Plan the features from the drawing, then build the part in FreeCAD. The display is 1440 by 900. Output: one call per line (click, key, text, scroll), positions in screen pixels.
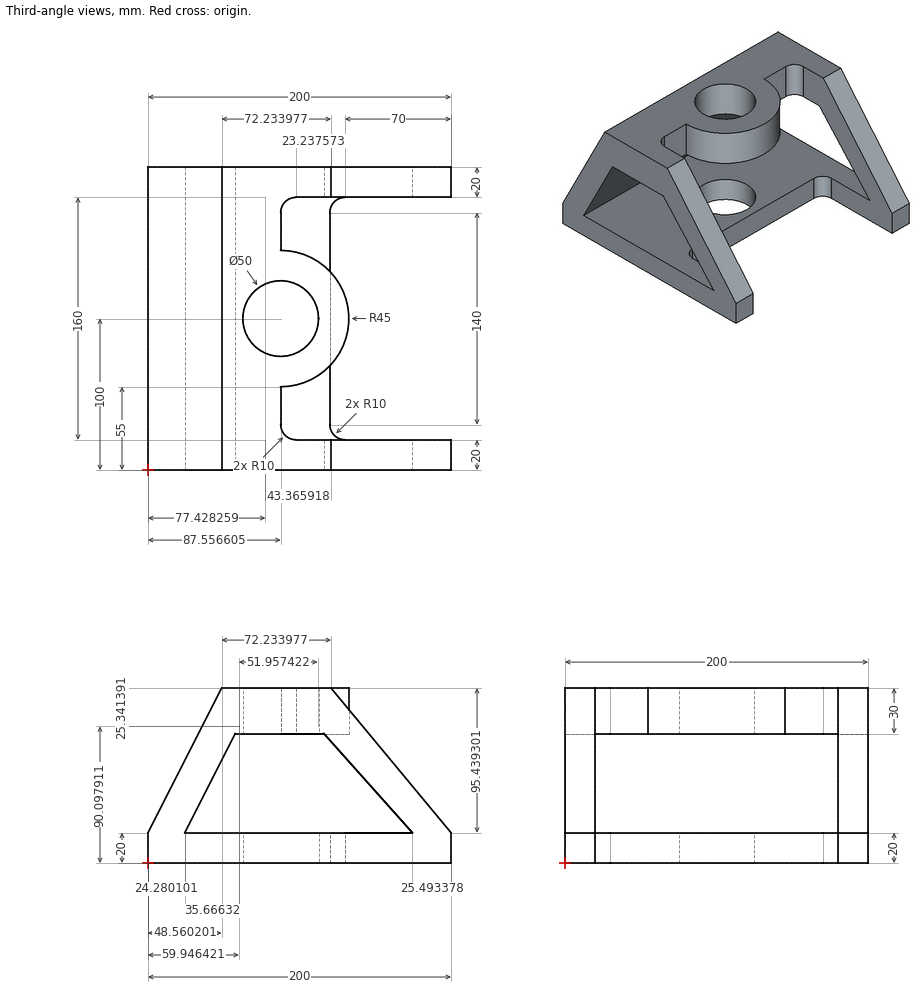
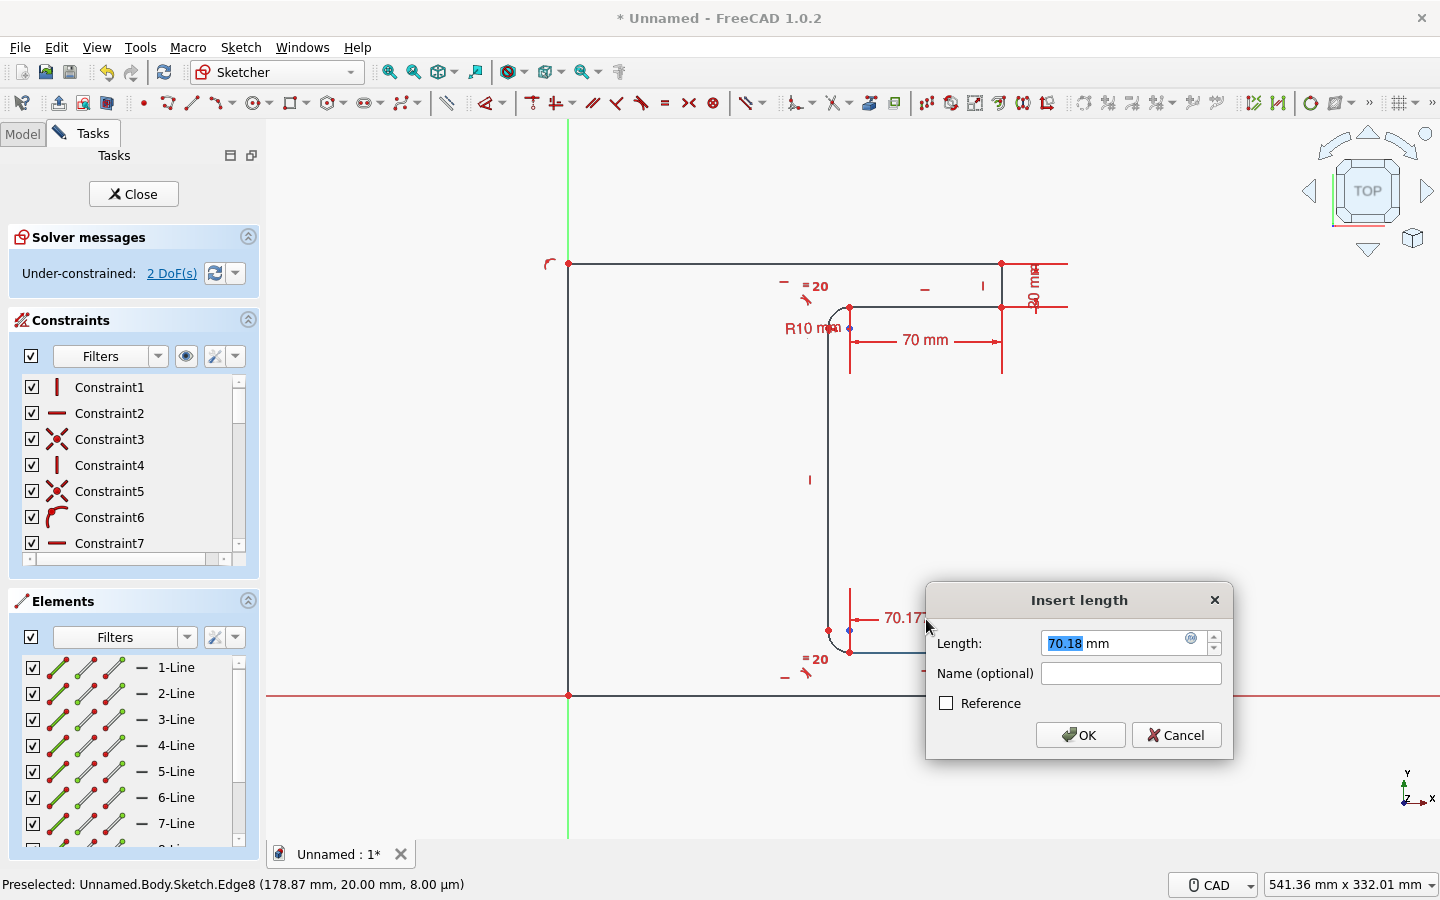
text(70)
key(Return)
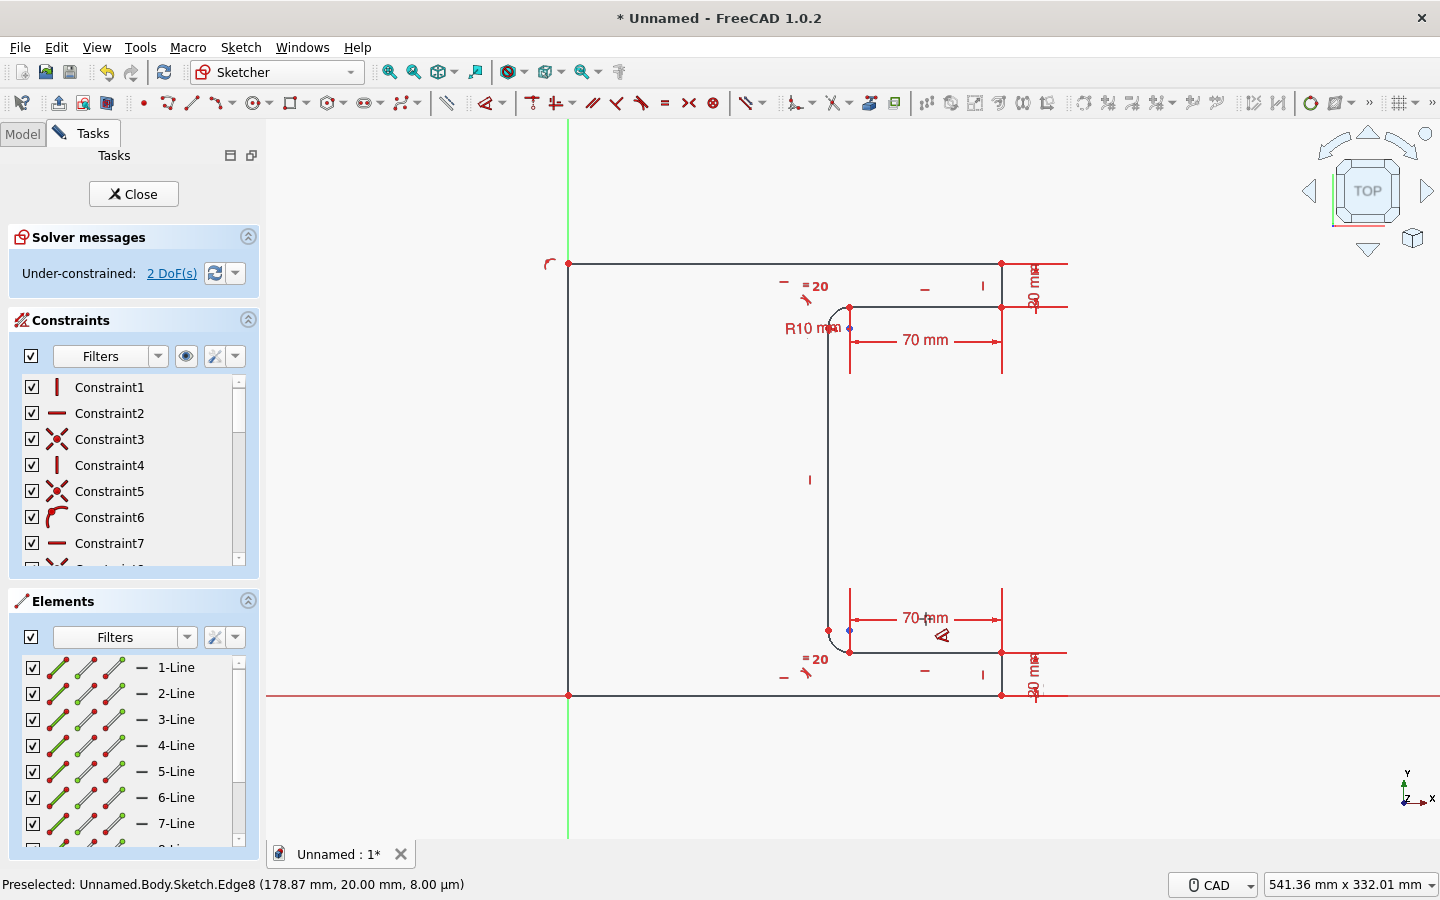
click(828, 540)
click(862, 480)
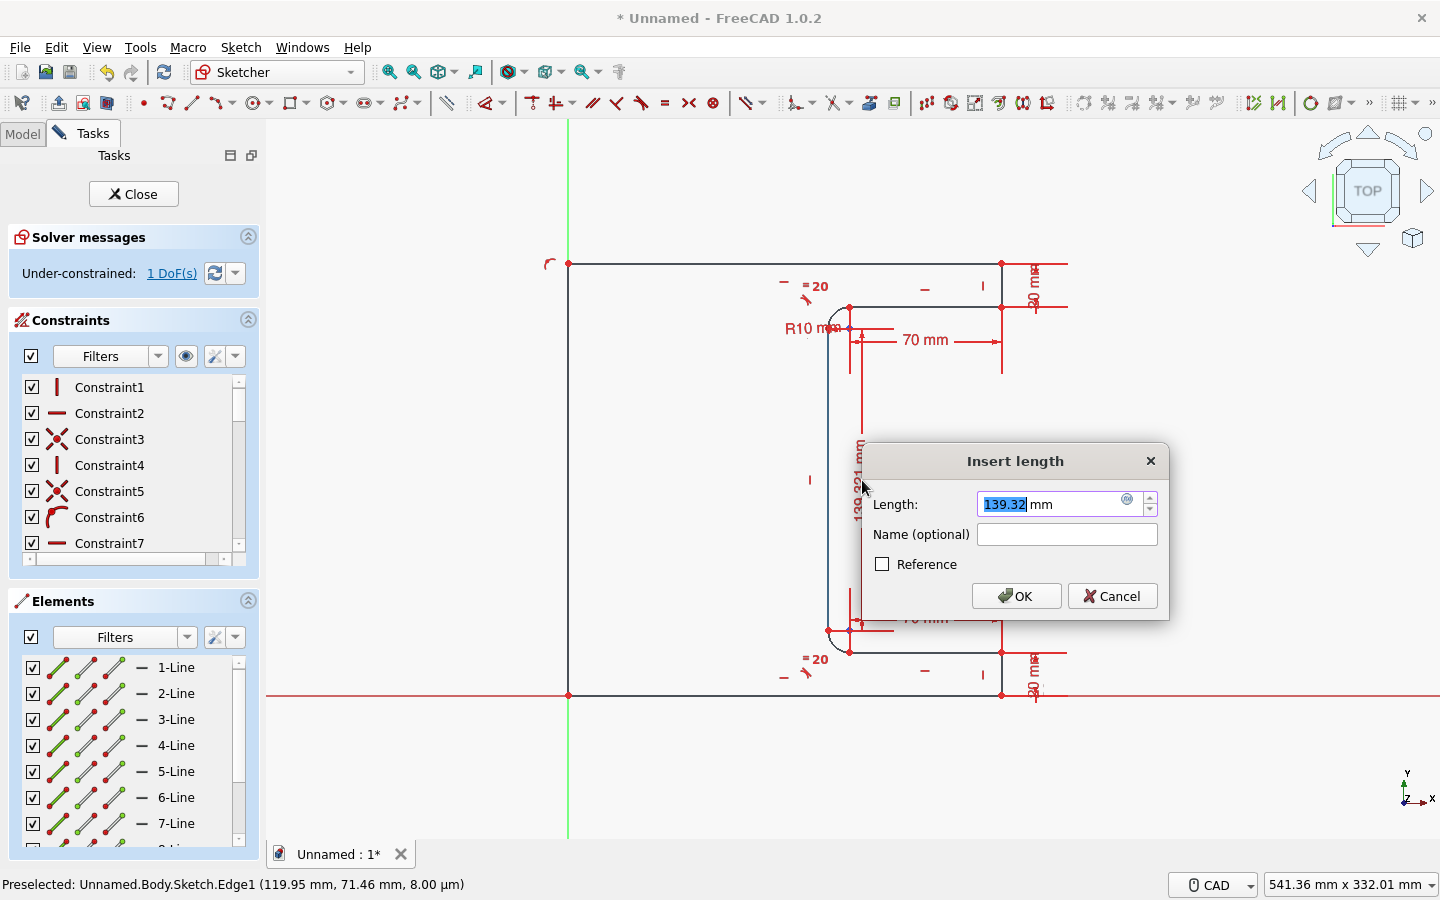
text(140)
key(Return)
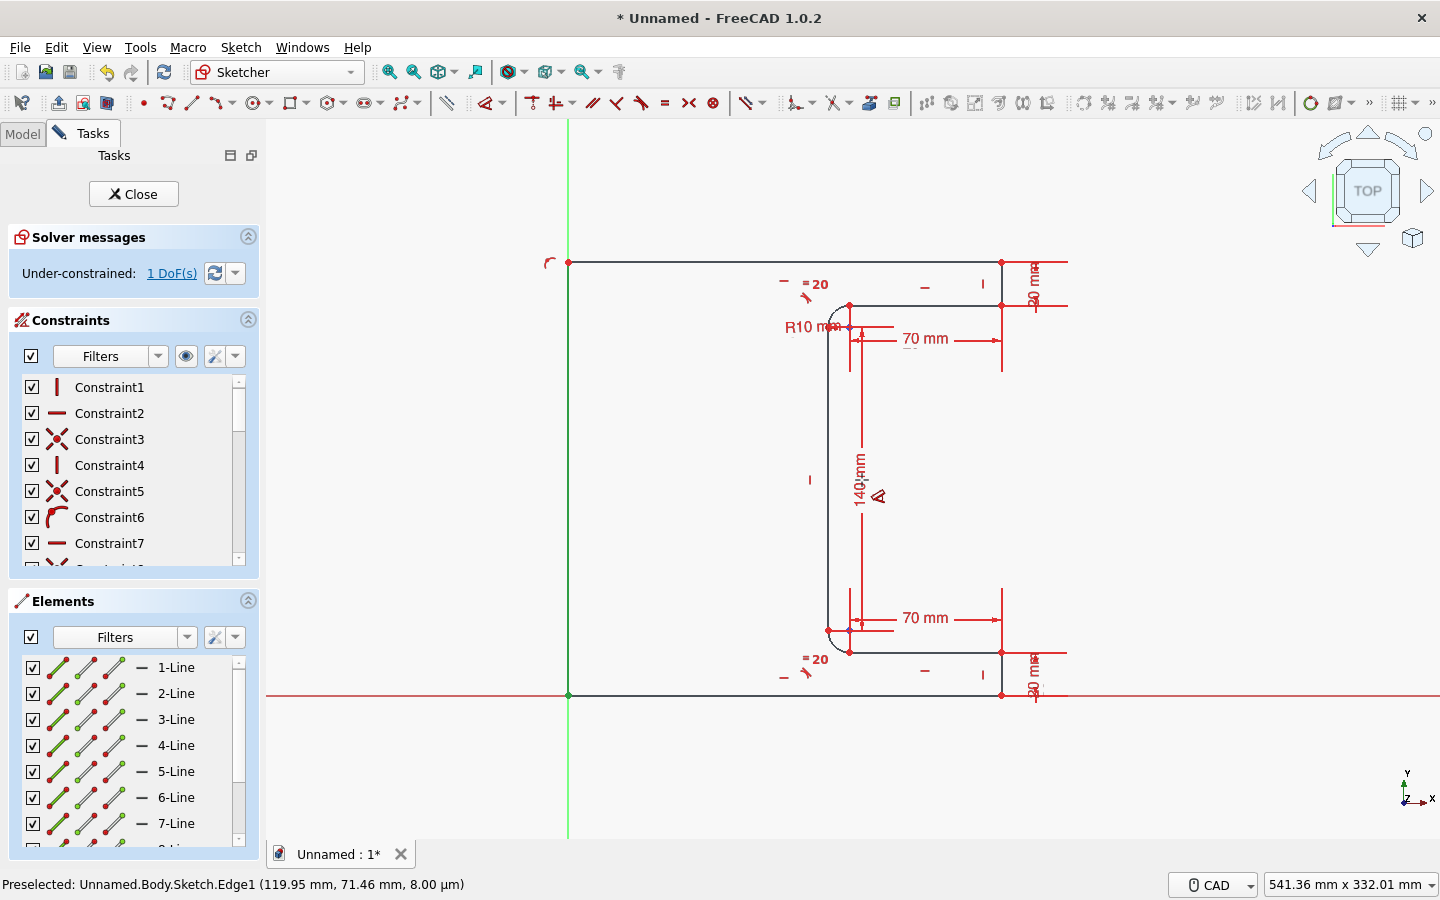
click(872, 262)
click(785, 228)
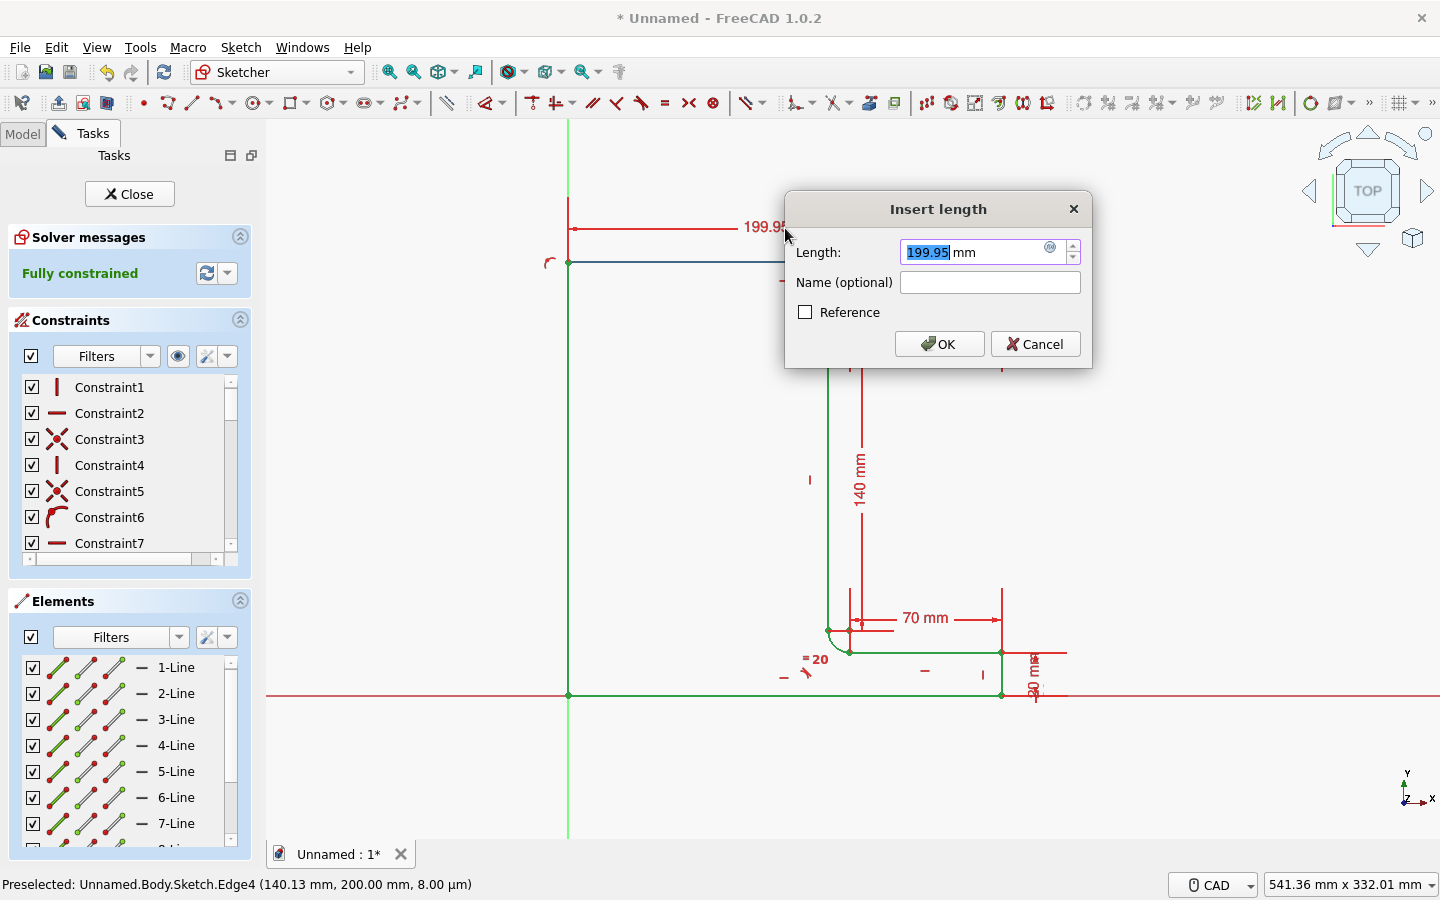
text(200)
key(Return)
key(Escape)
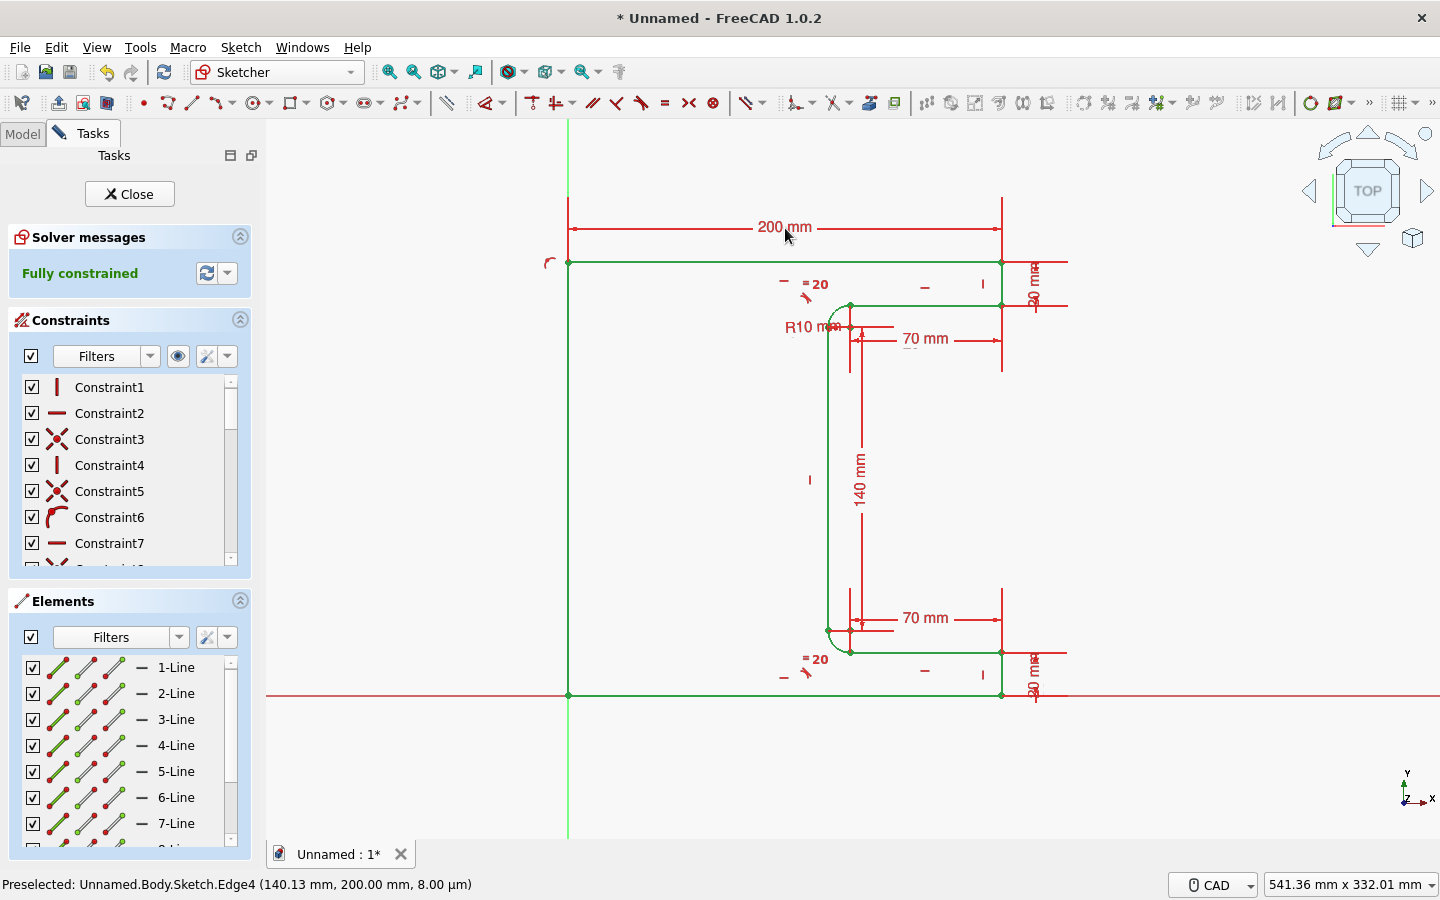
click(130, 194)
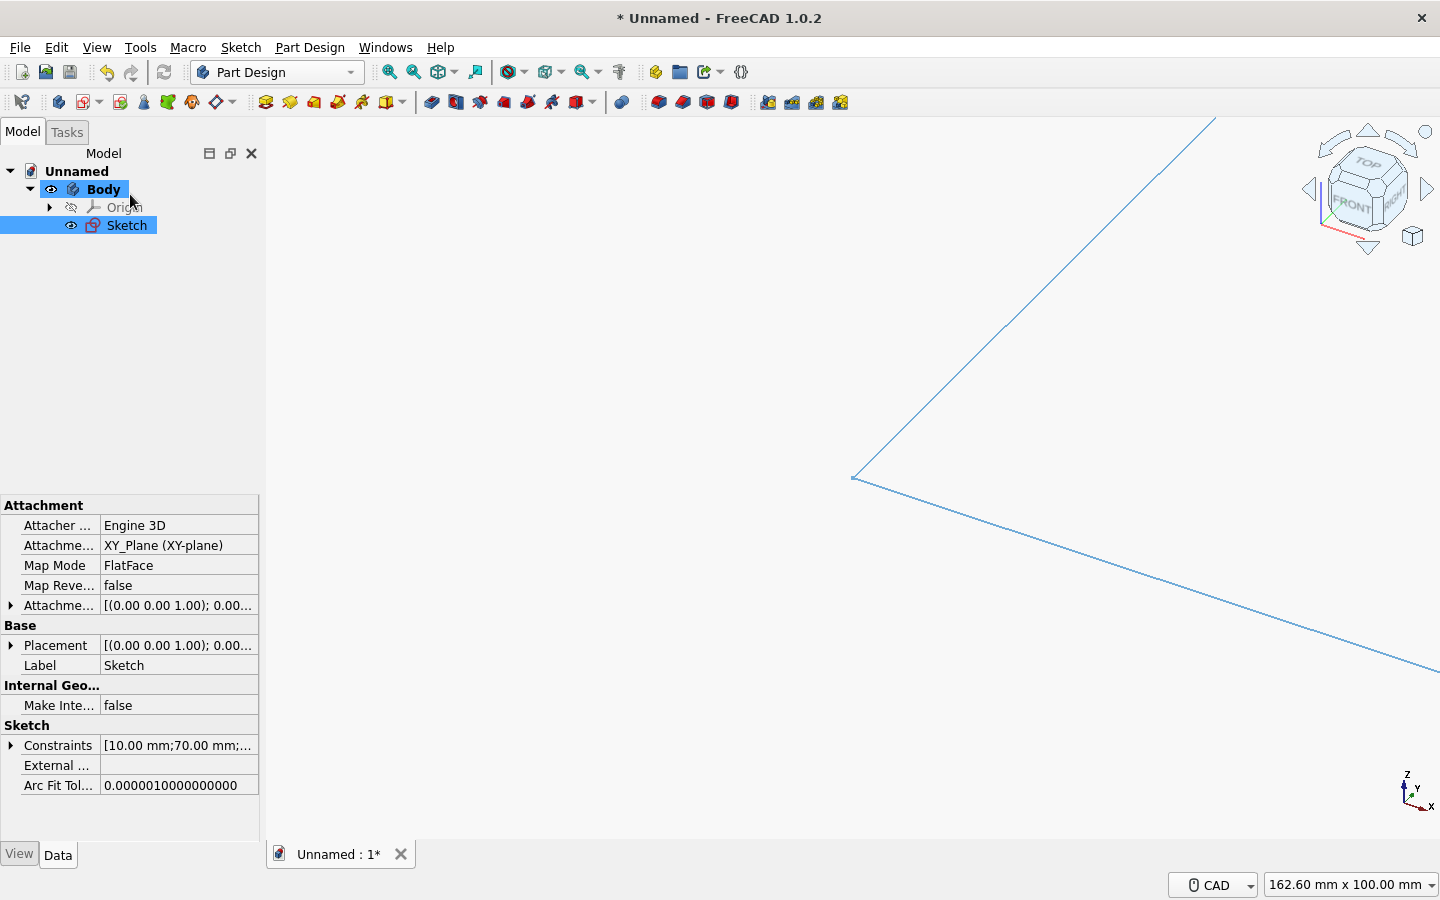
click(266, 102)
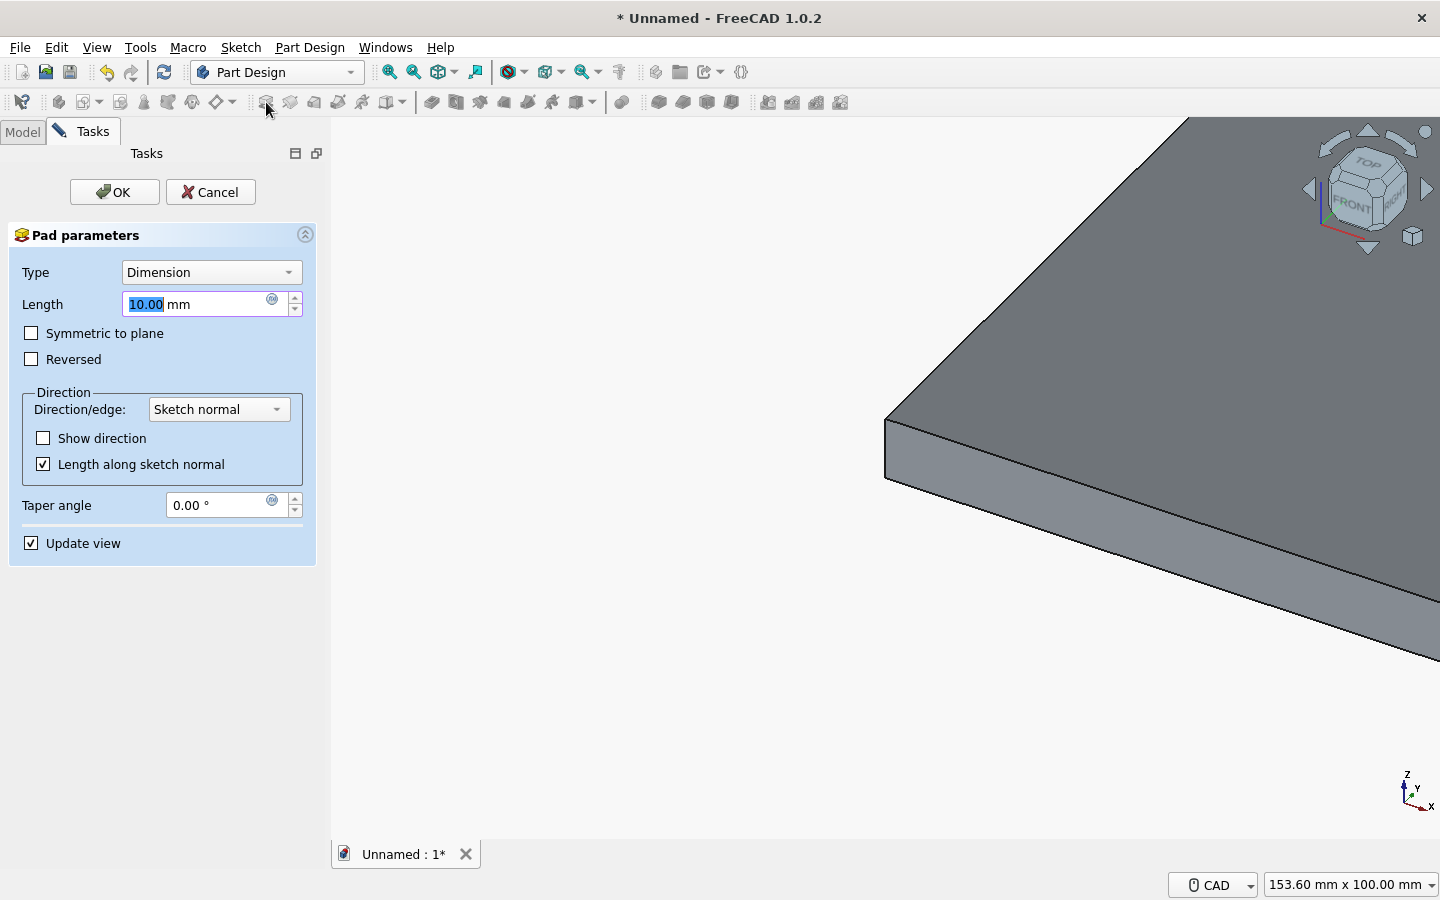
text(20)
key(Tab)